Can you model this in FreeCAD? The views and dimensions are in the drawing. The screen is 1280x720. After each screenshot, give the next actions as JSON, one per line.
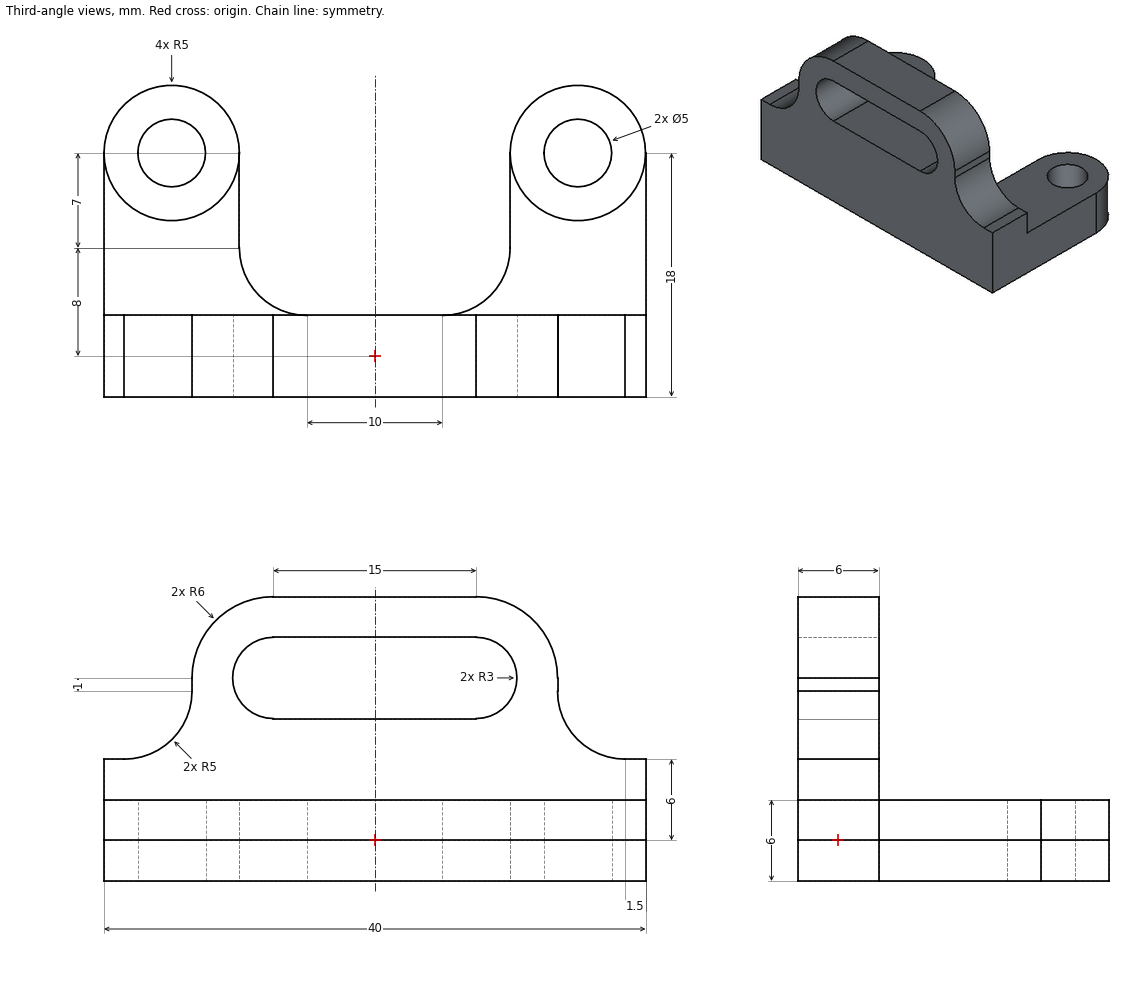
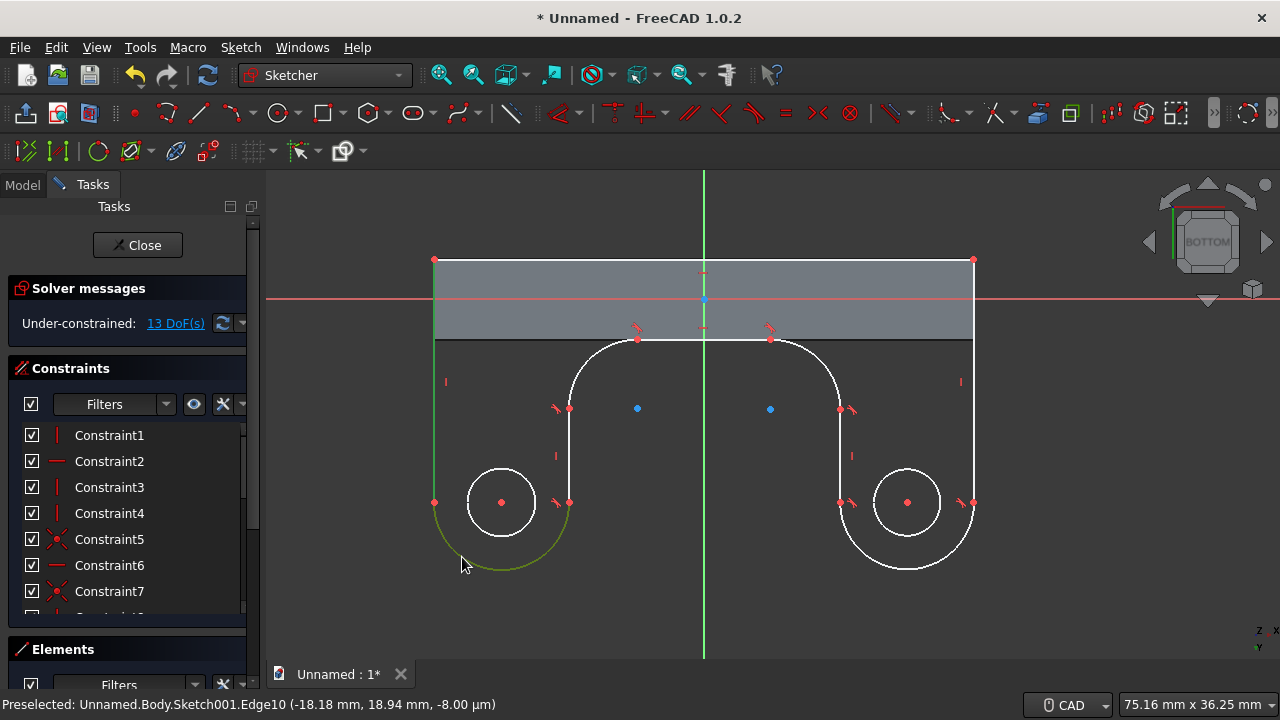
{"action": "key", "text": "t"}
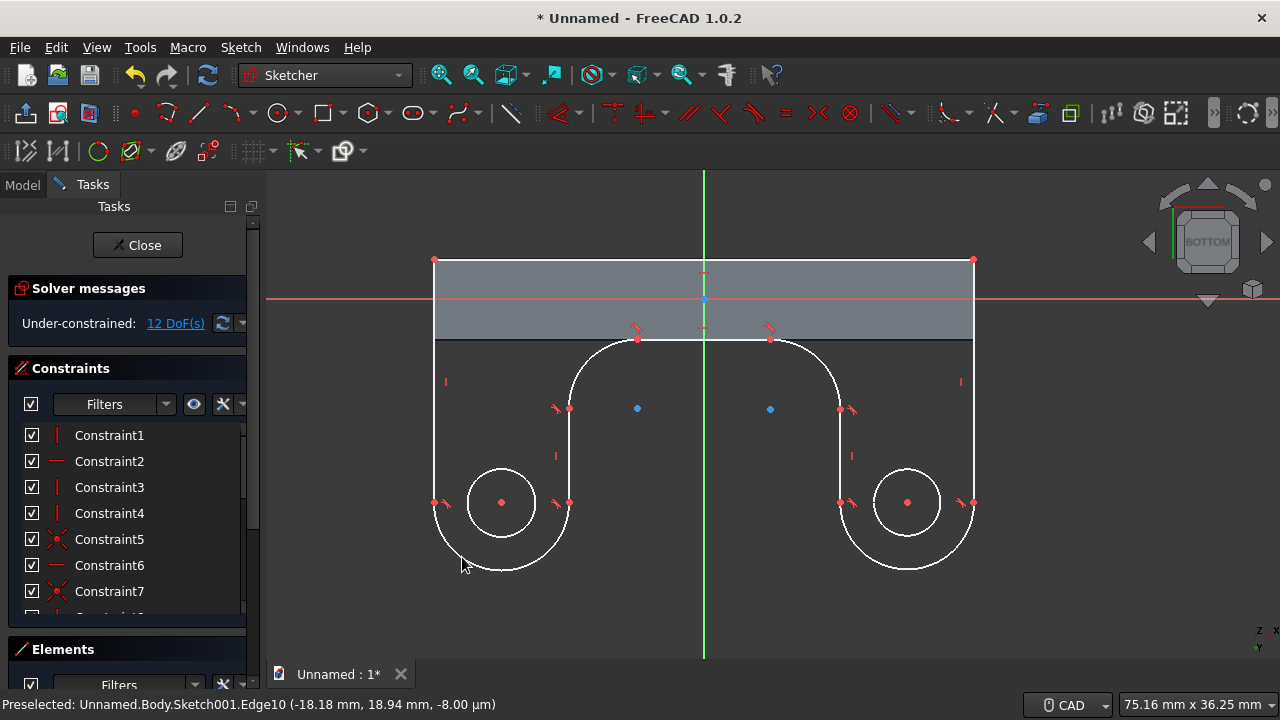
{"action": "left_click", "coordinate": [606, 347]}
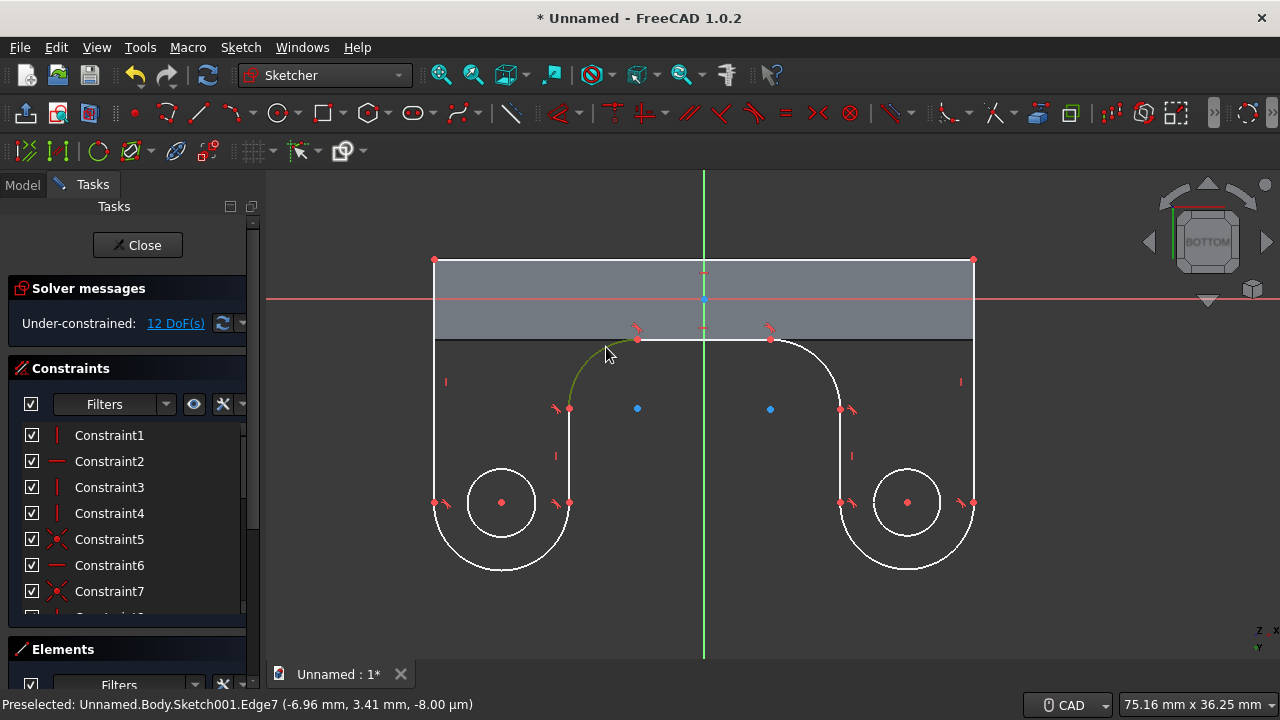
{"action": "left_click", "coordinate": [833, 378]}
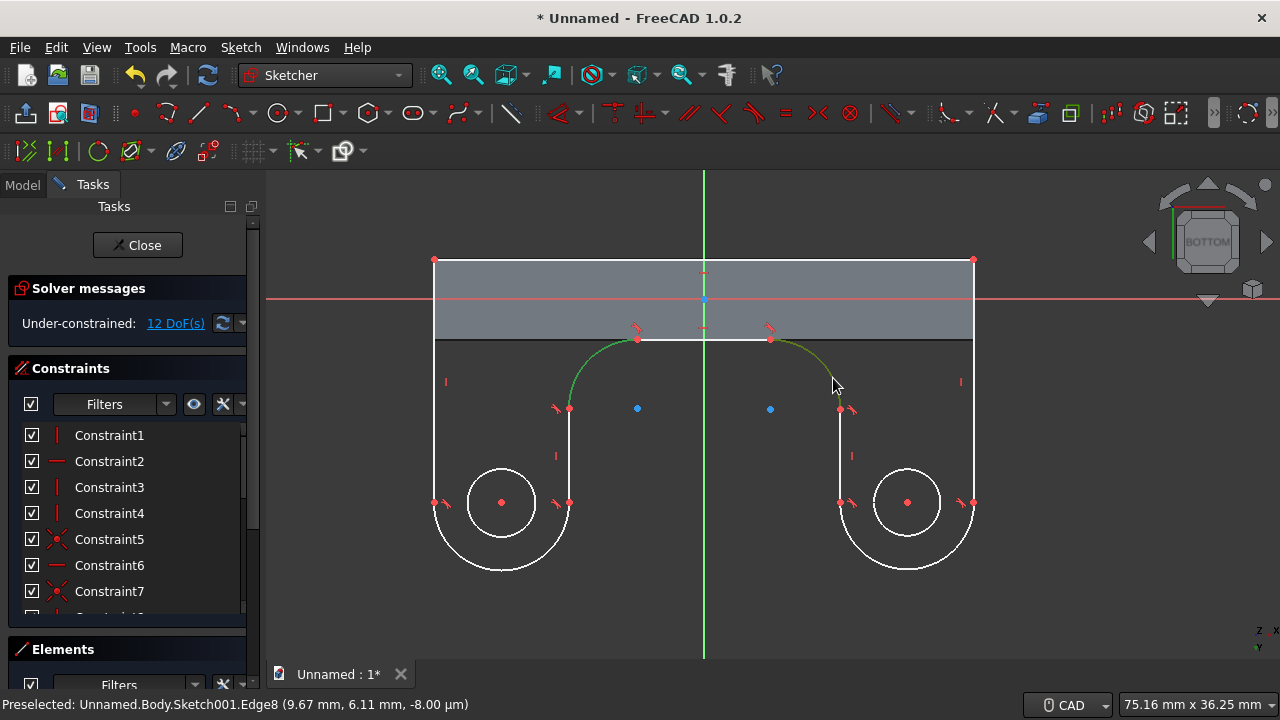
{"action": "left_click", "coordinate": [868, 557]}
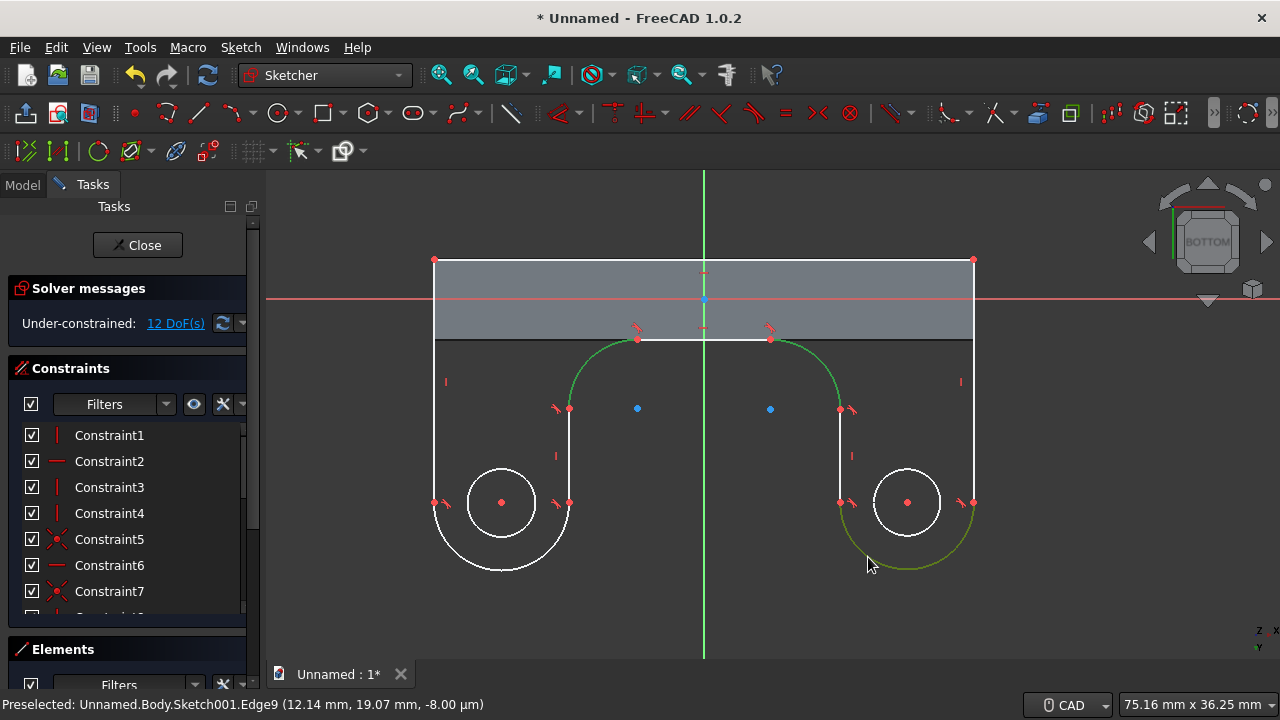
{"action": "left_click", "coordinate": [462, 558]}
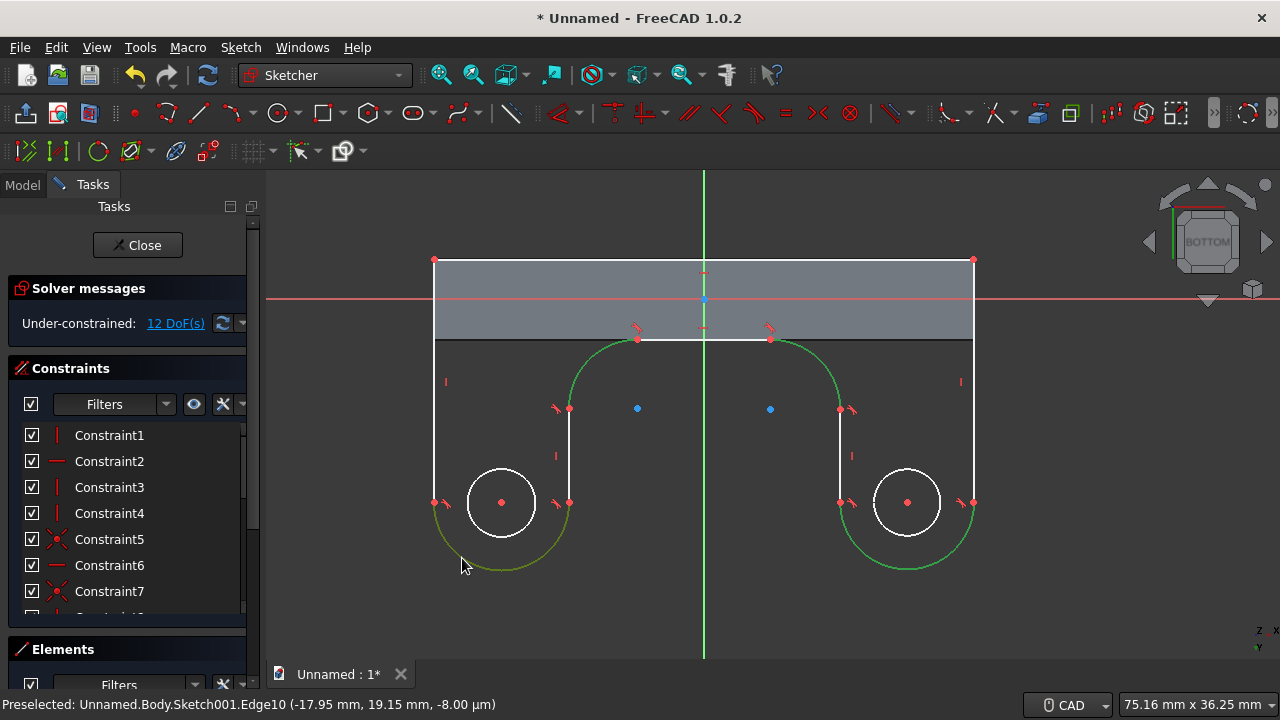
{"action": "left_click", "coordinate": [786, 114]}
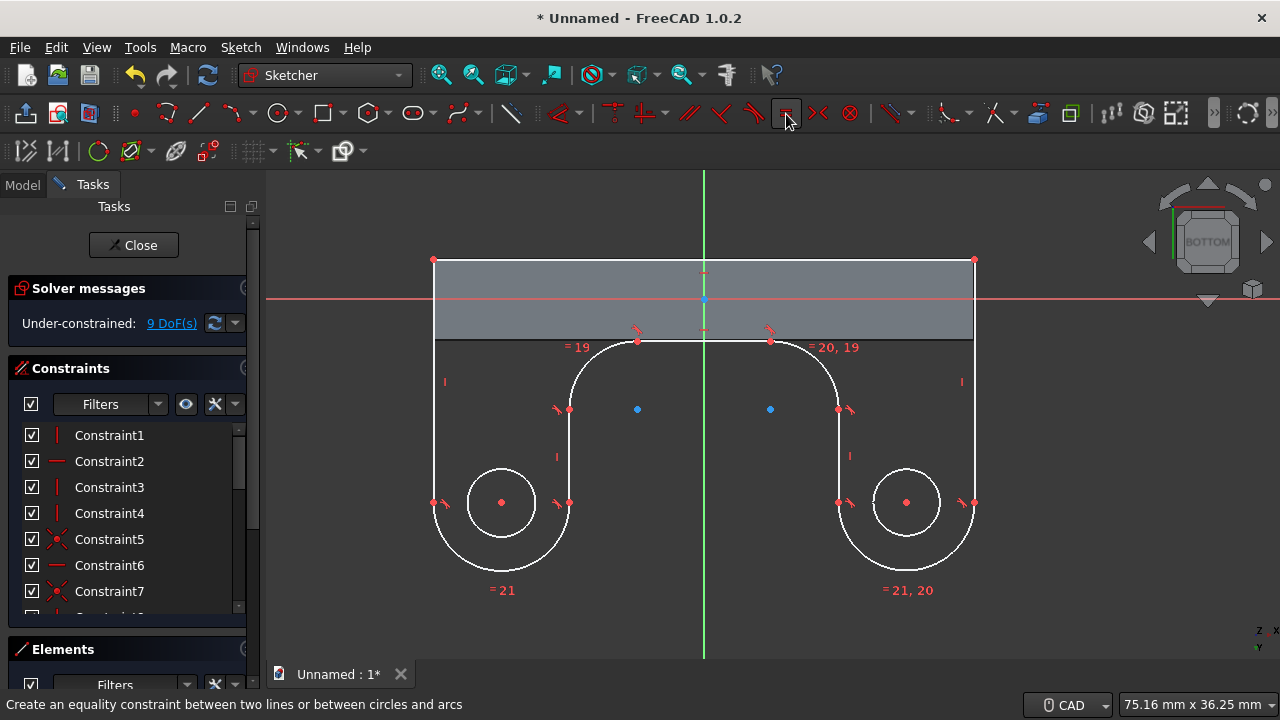
{"action": "left_click", "coordinate": [930, 479]}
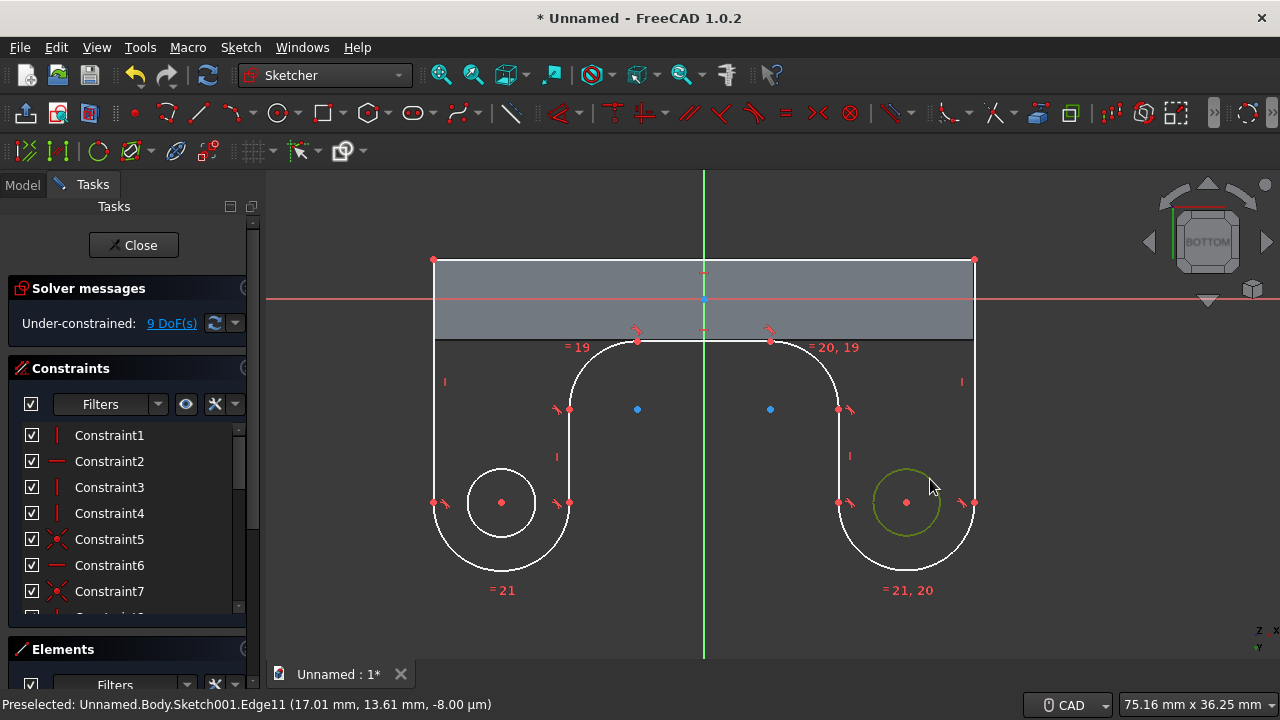
{"action": "left_click", "coordinate": [525, 479]}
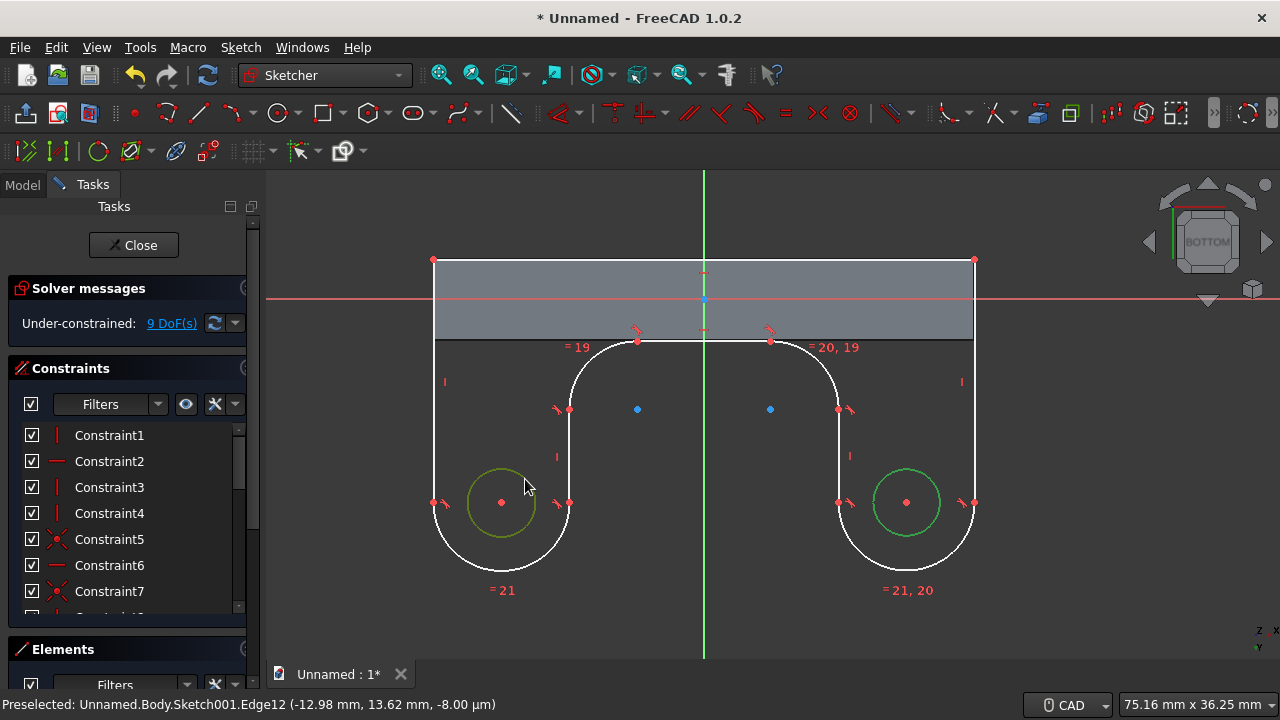
{"action": "key", "text": "e"}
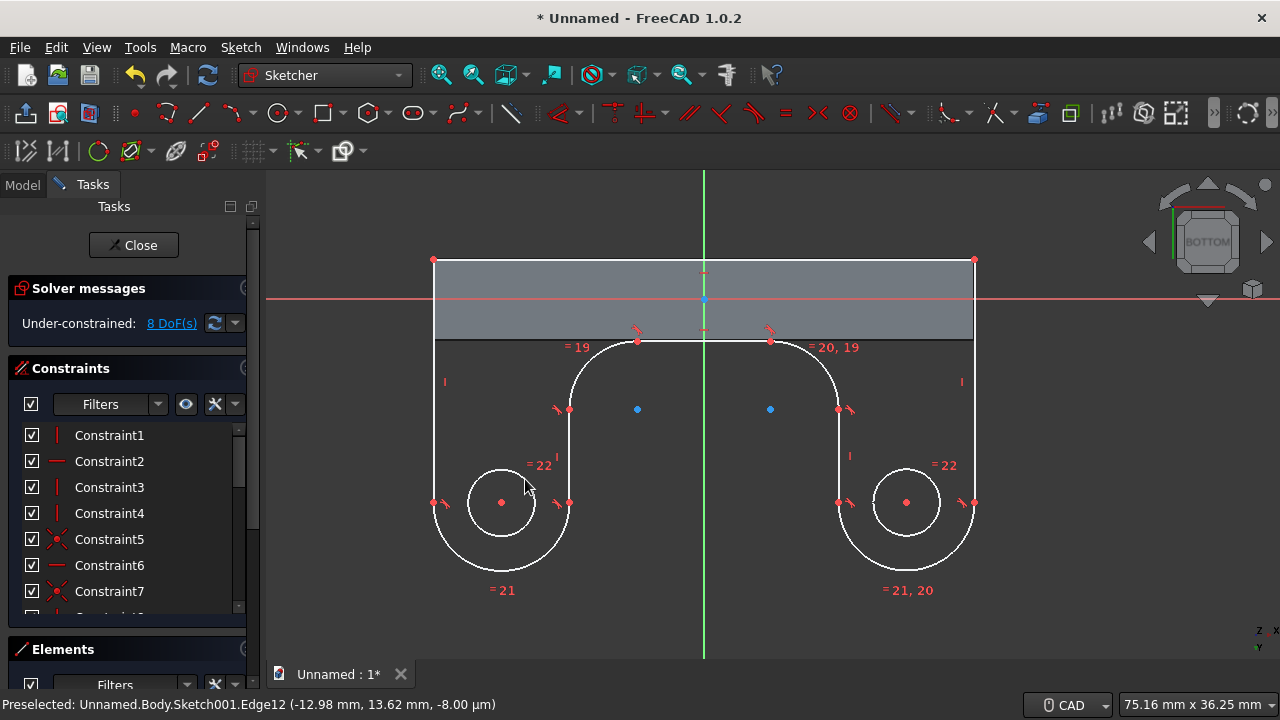
{"action": "left_click", "coordinate": [907, 503]}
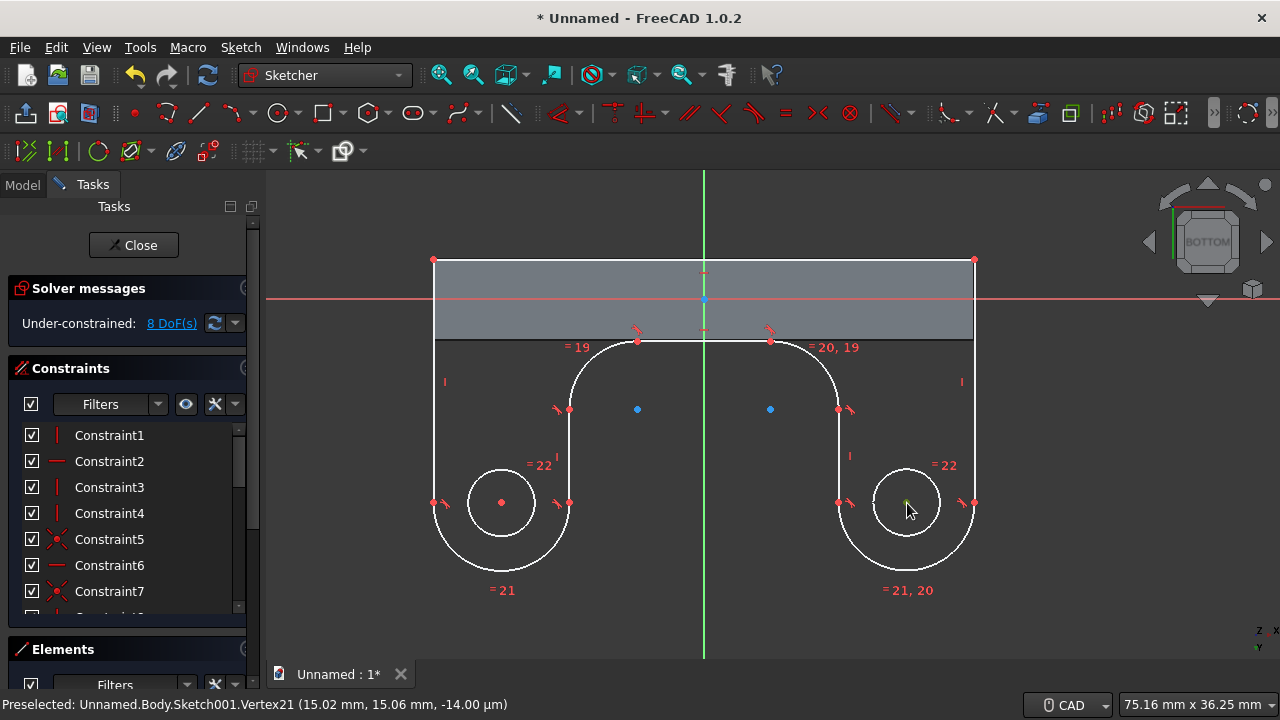
{"action": "left_click", "coordinate": [501, 503]}